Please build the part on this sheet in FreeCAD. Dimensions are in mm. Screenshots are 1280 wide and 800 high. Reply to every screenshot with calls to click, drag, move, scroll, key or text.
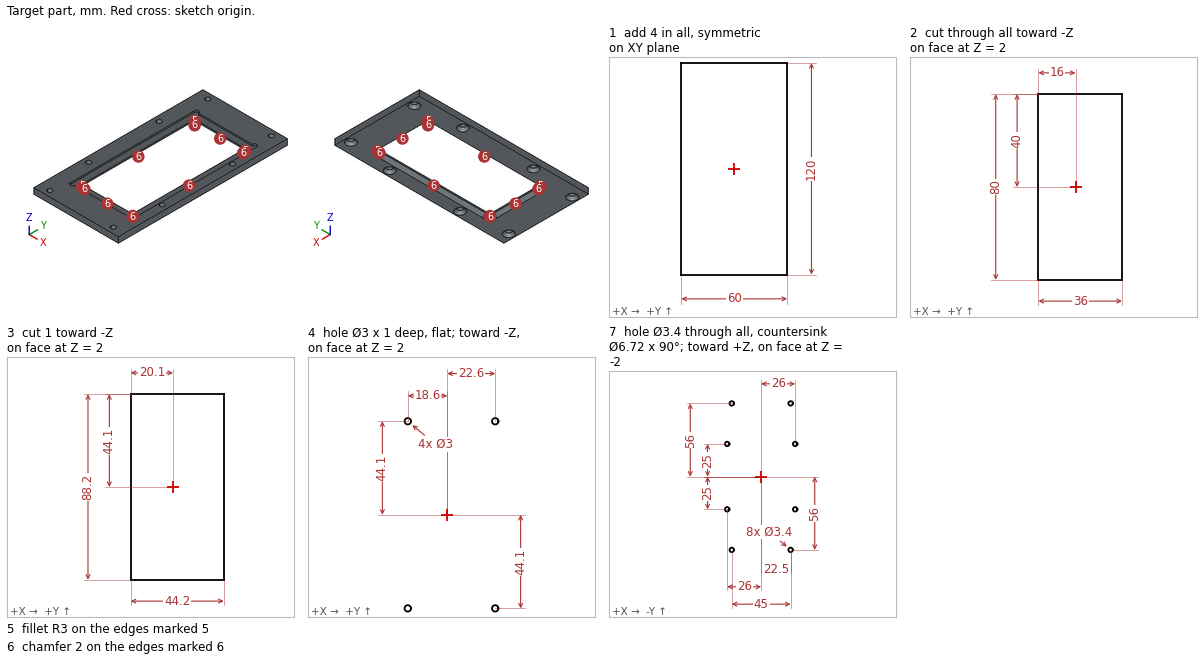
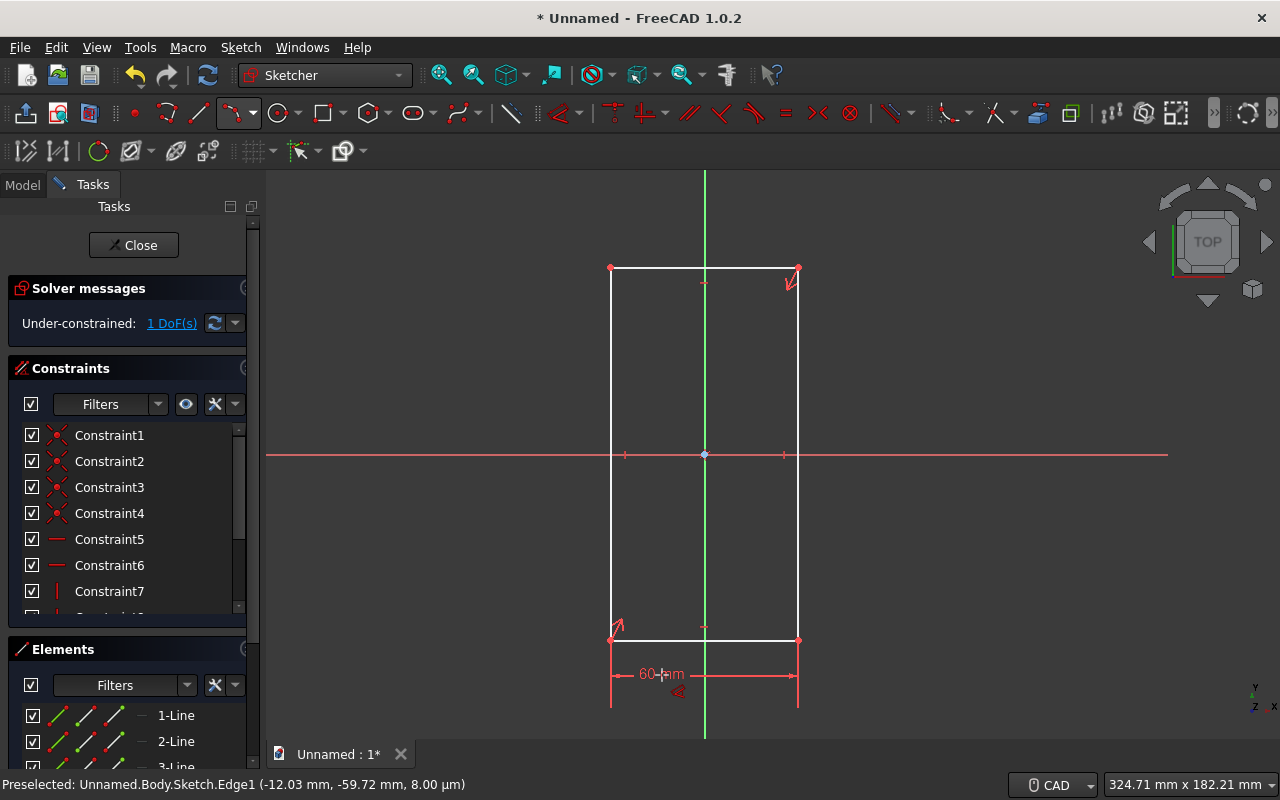
click(798, 529)
click(832, 369)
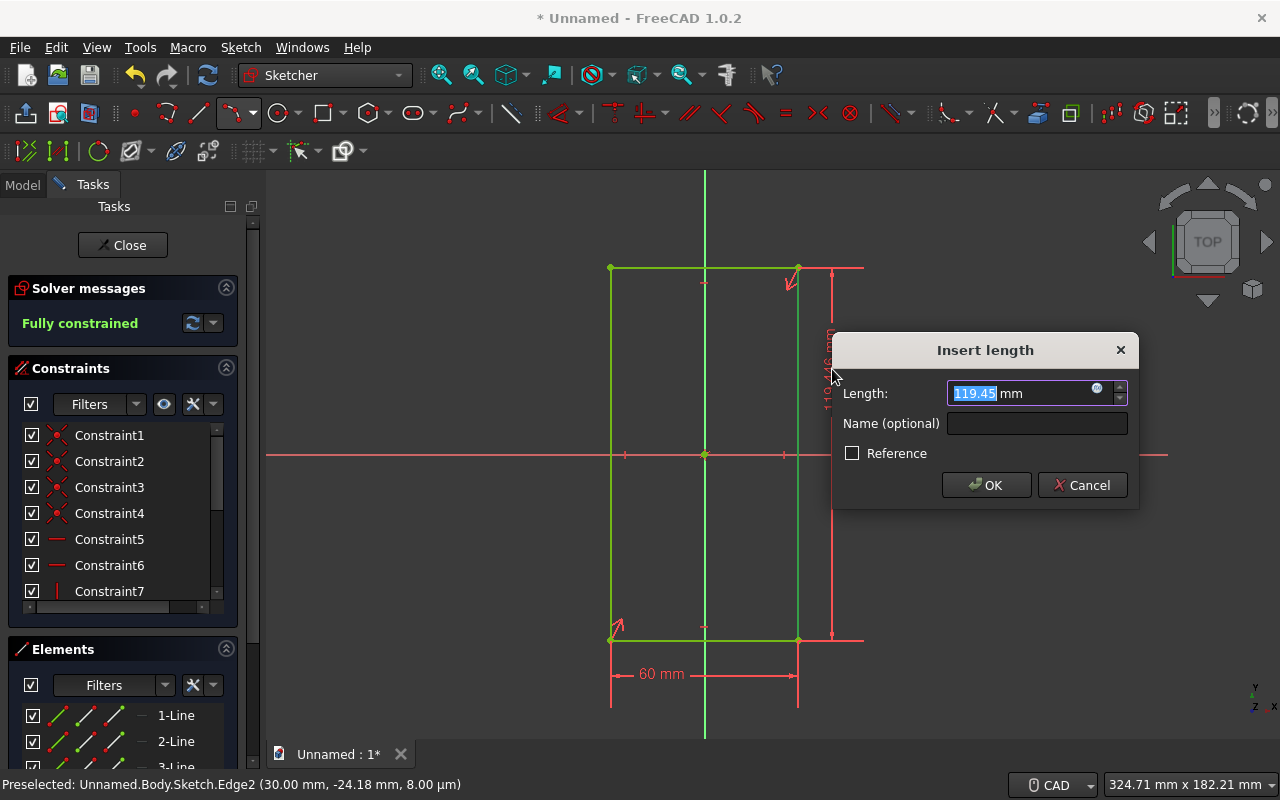
text(120)
key(Return)
key(Escape)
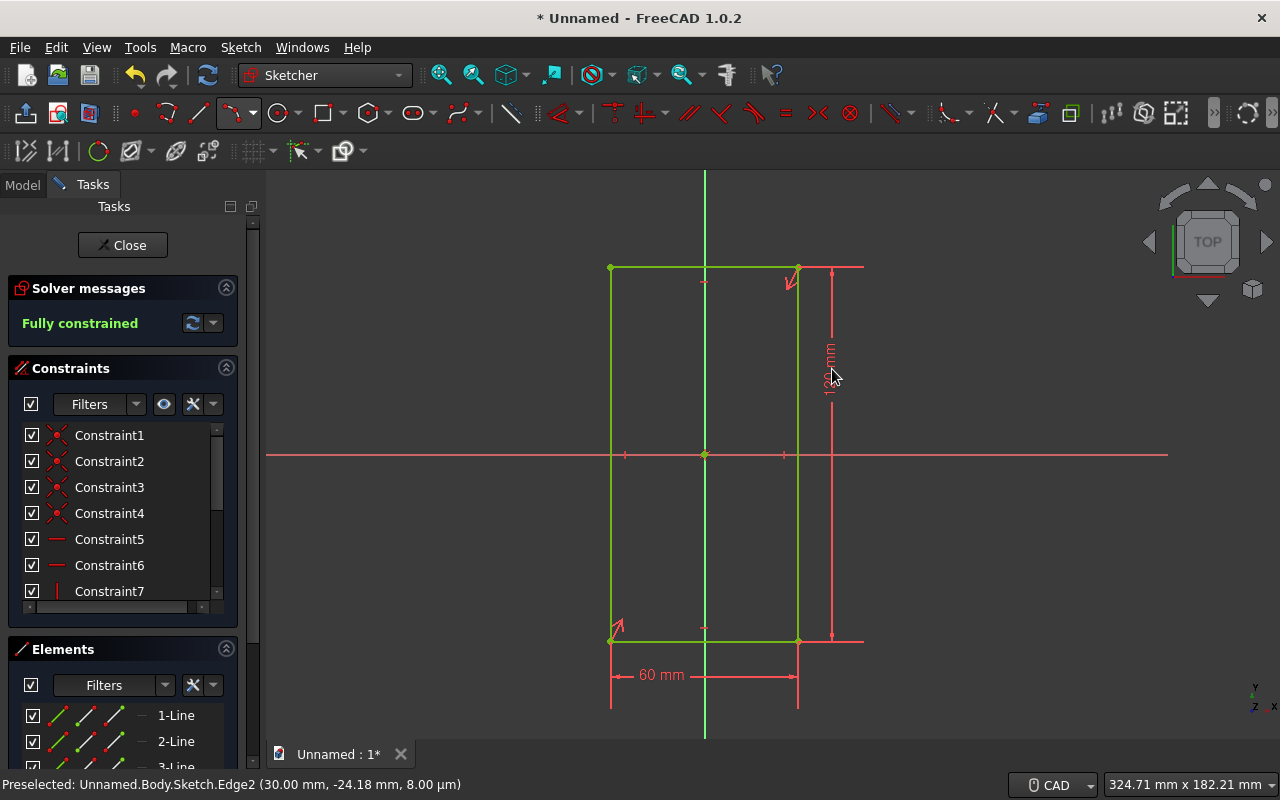
click(123, 245)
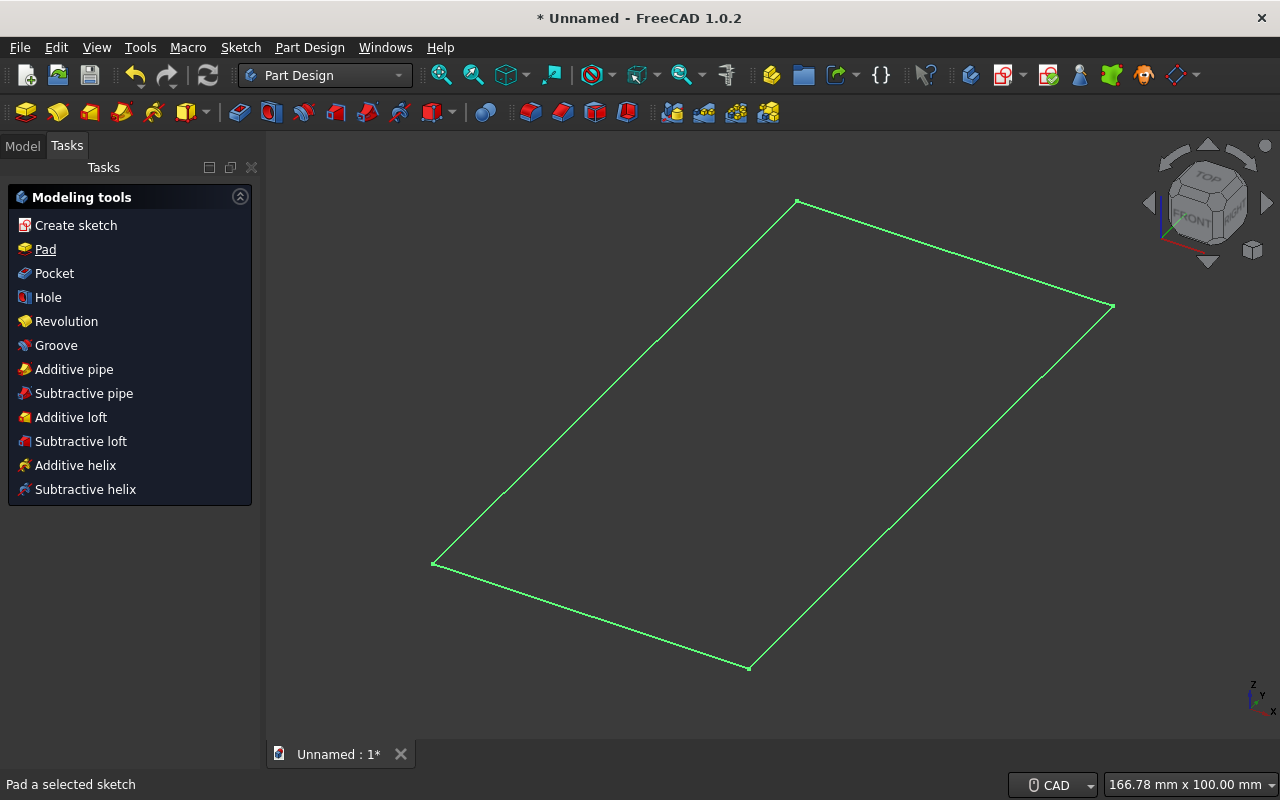
click(26, 112)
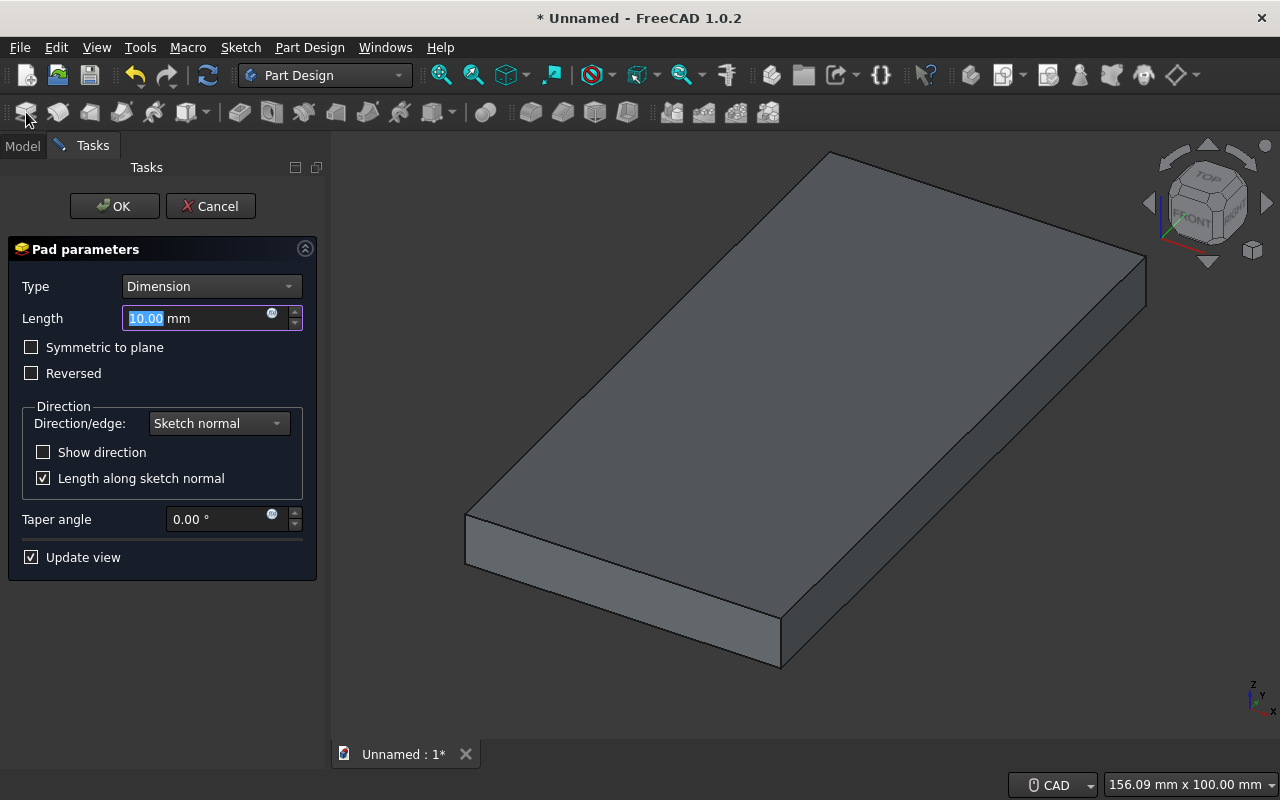
text(4)
key(Tab)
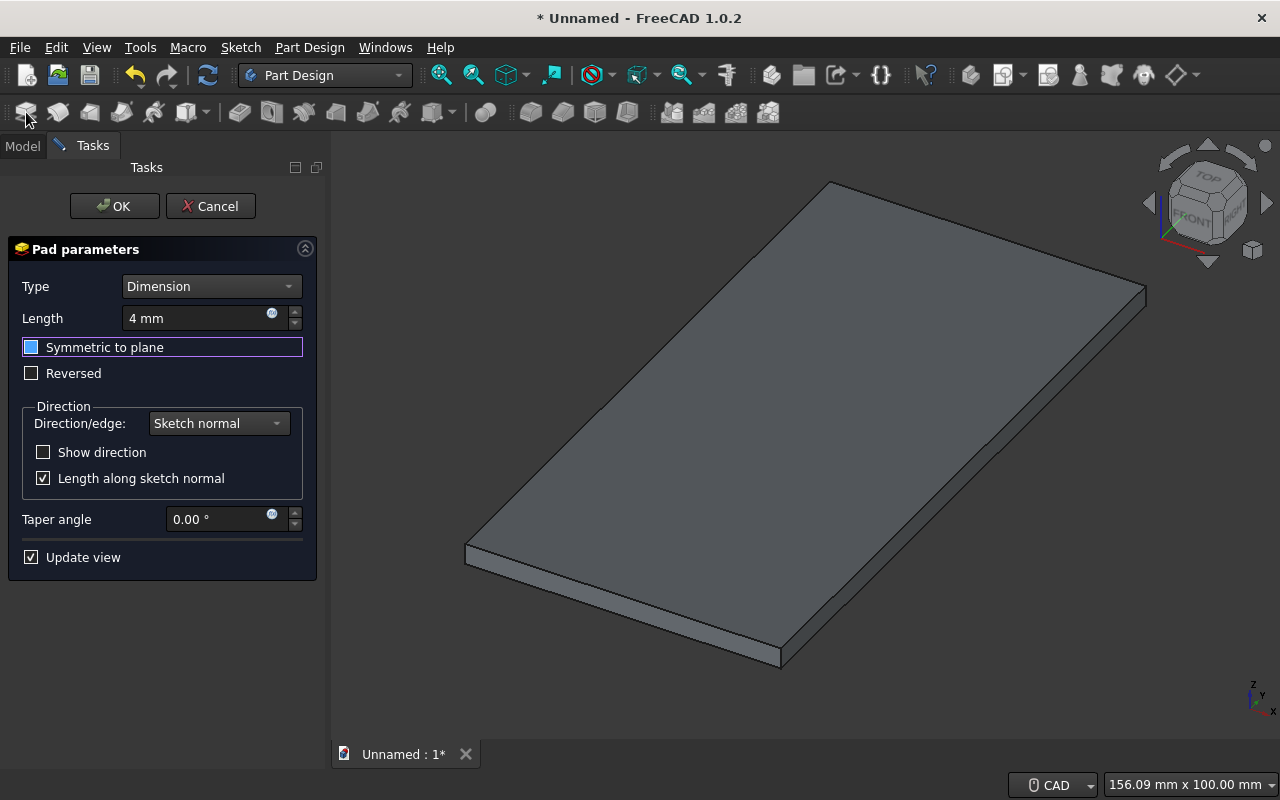
click(30, 347)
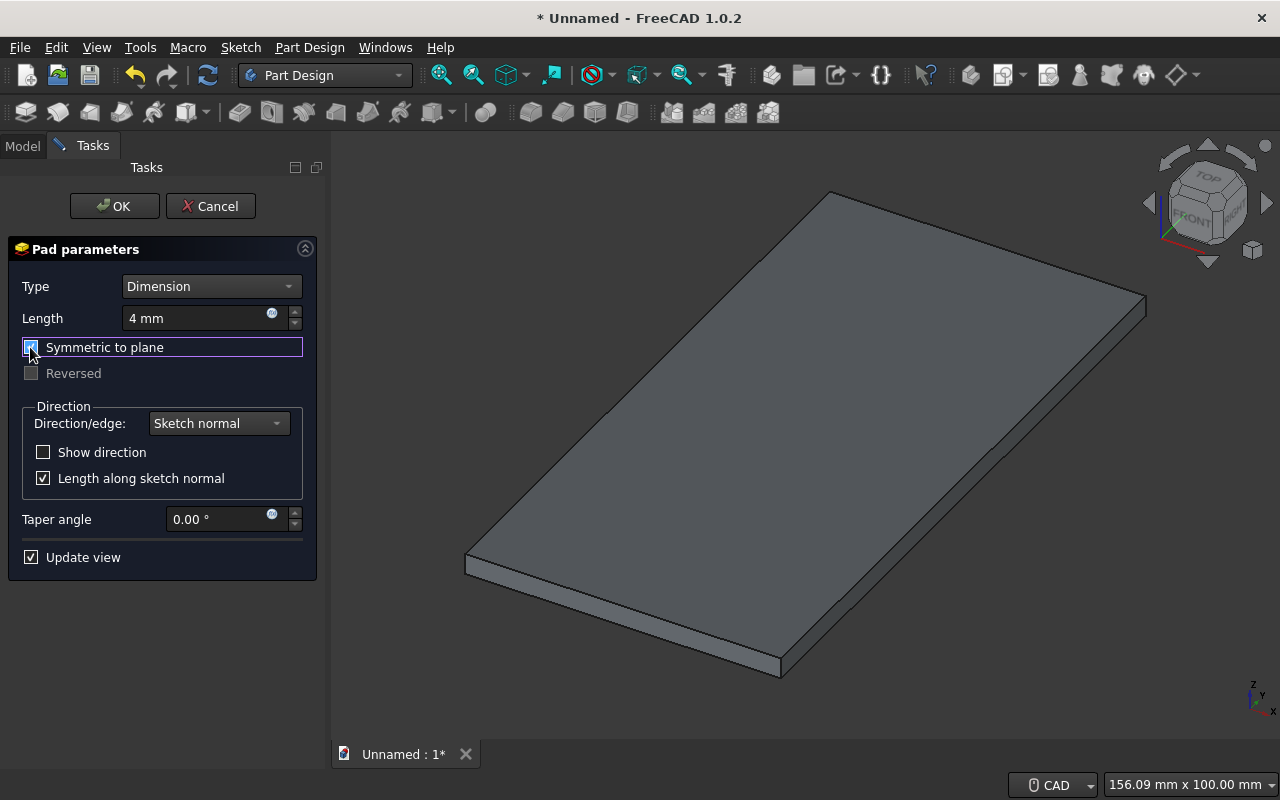
click(115, 206)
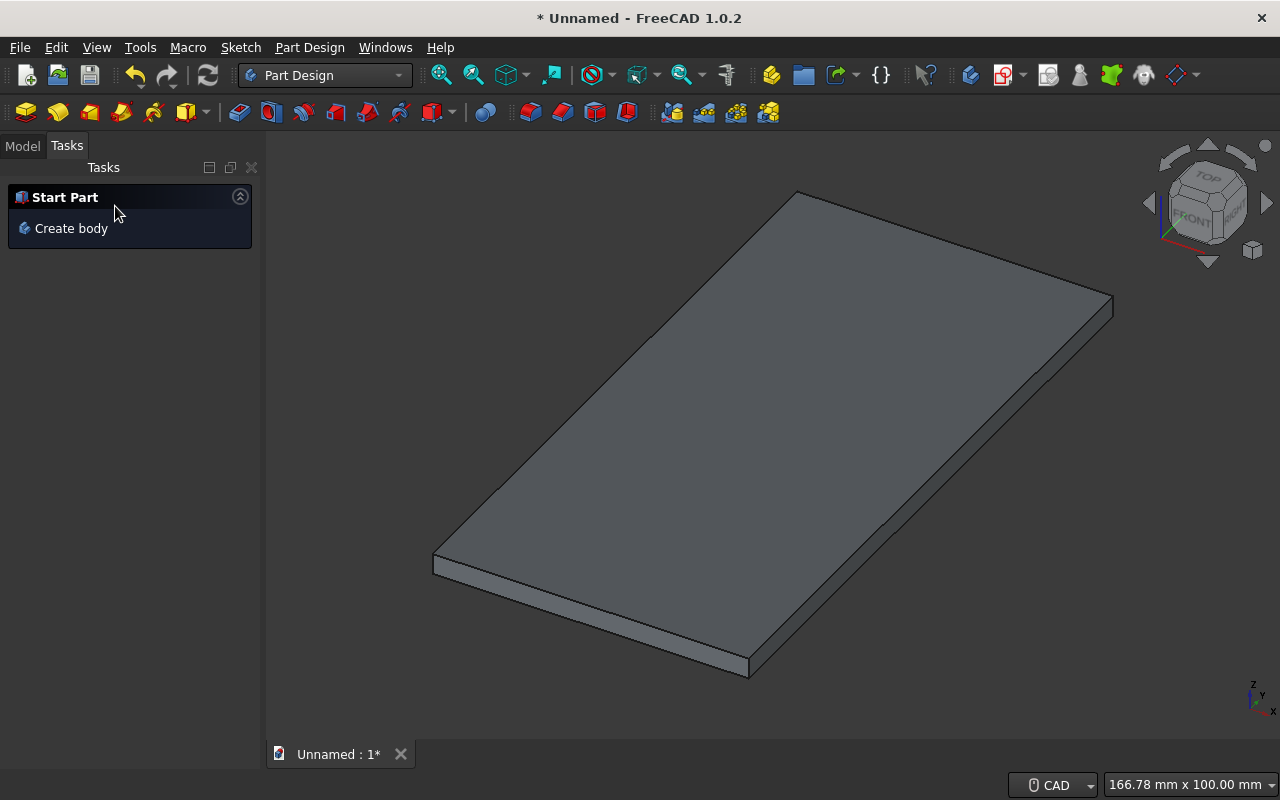
click(825, 372)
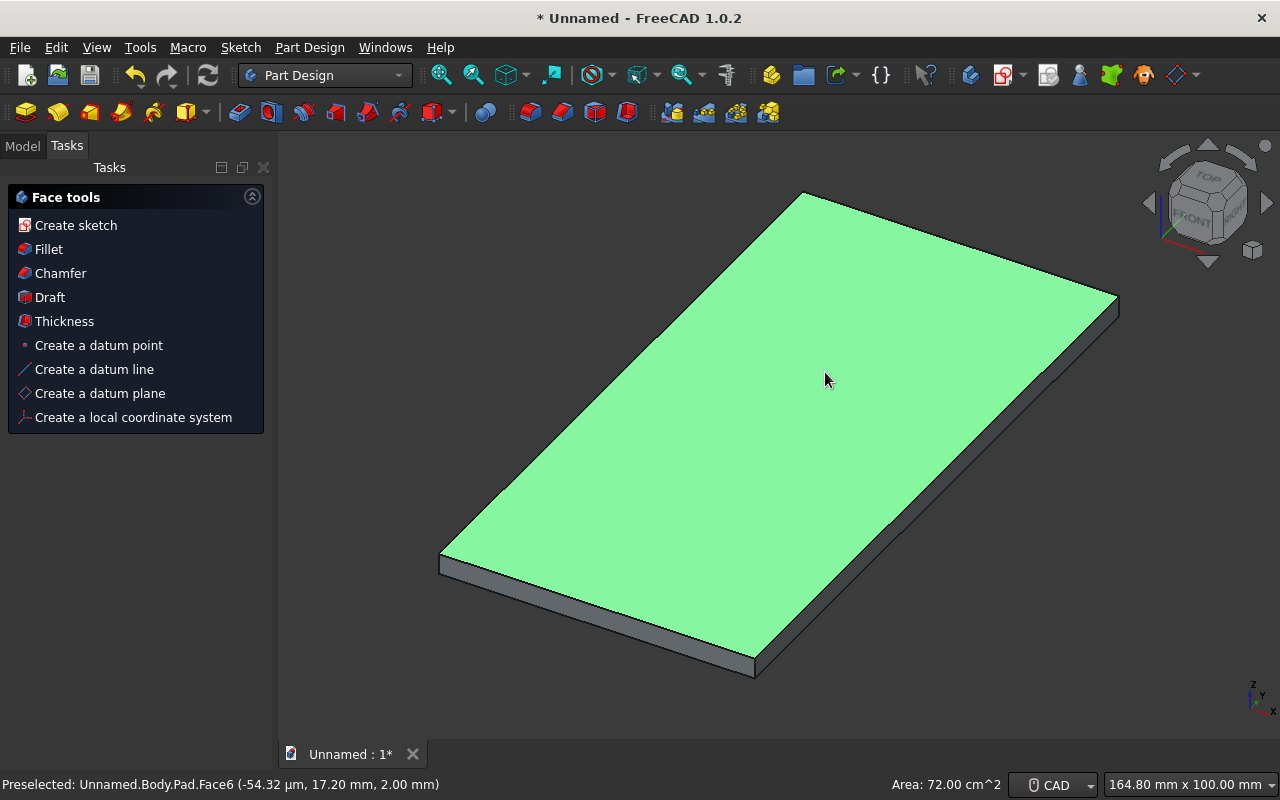
click(1004, 76)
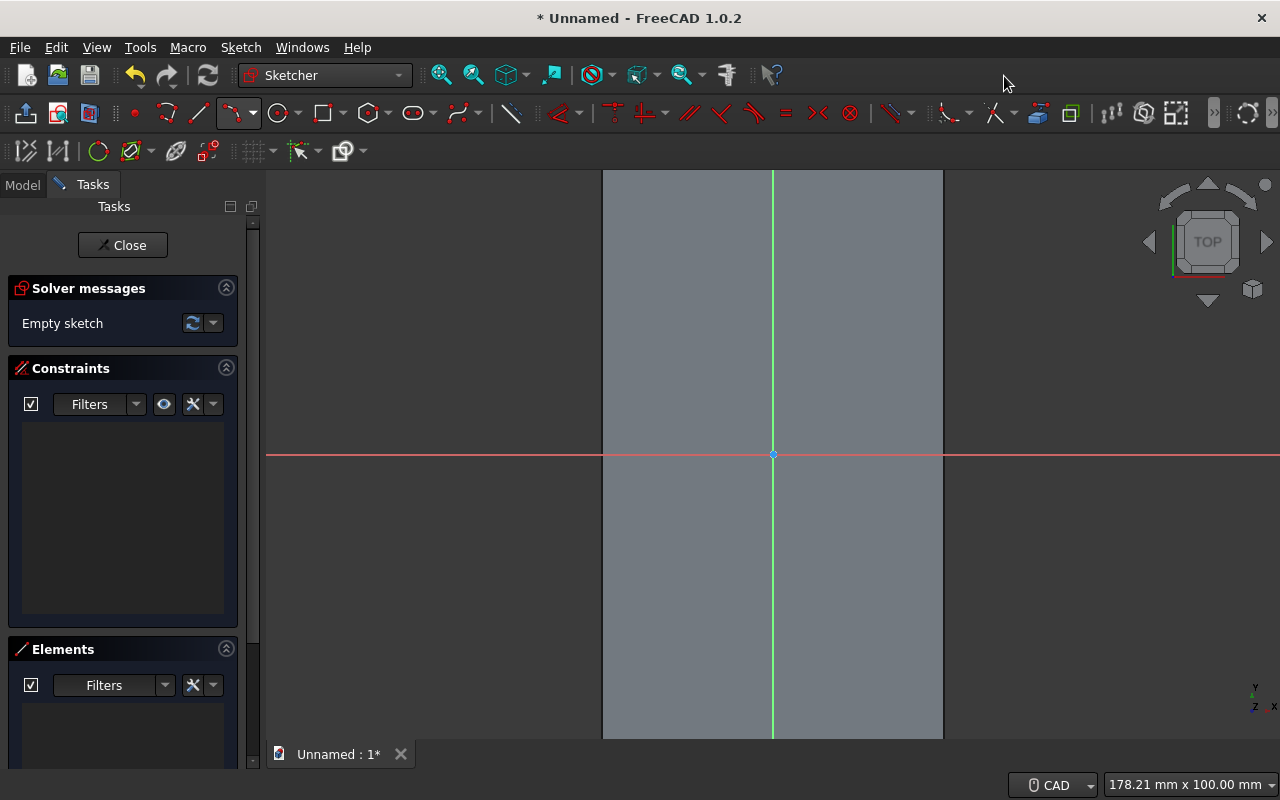
click(324, 114)